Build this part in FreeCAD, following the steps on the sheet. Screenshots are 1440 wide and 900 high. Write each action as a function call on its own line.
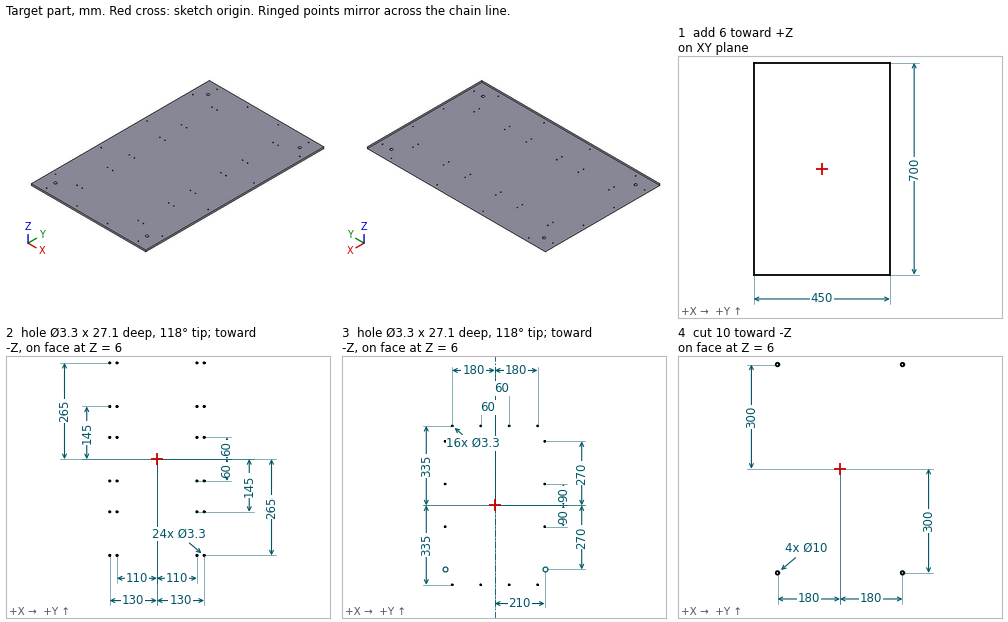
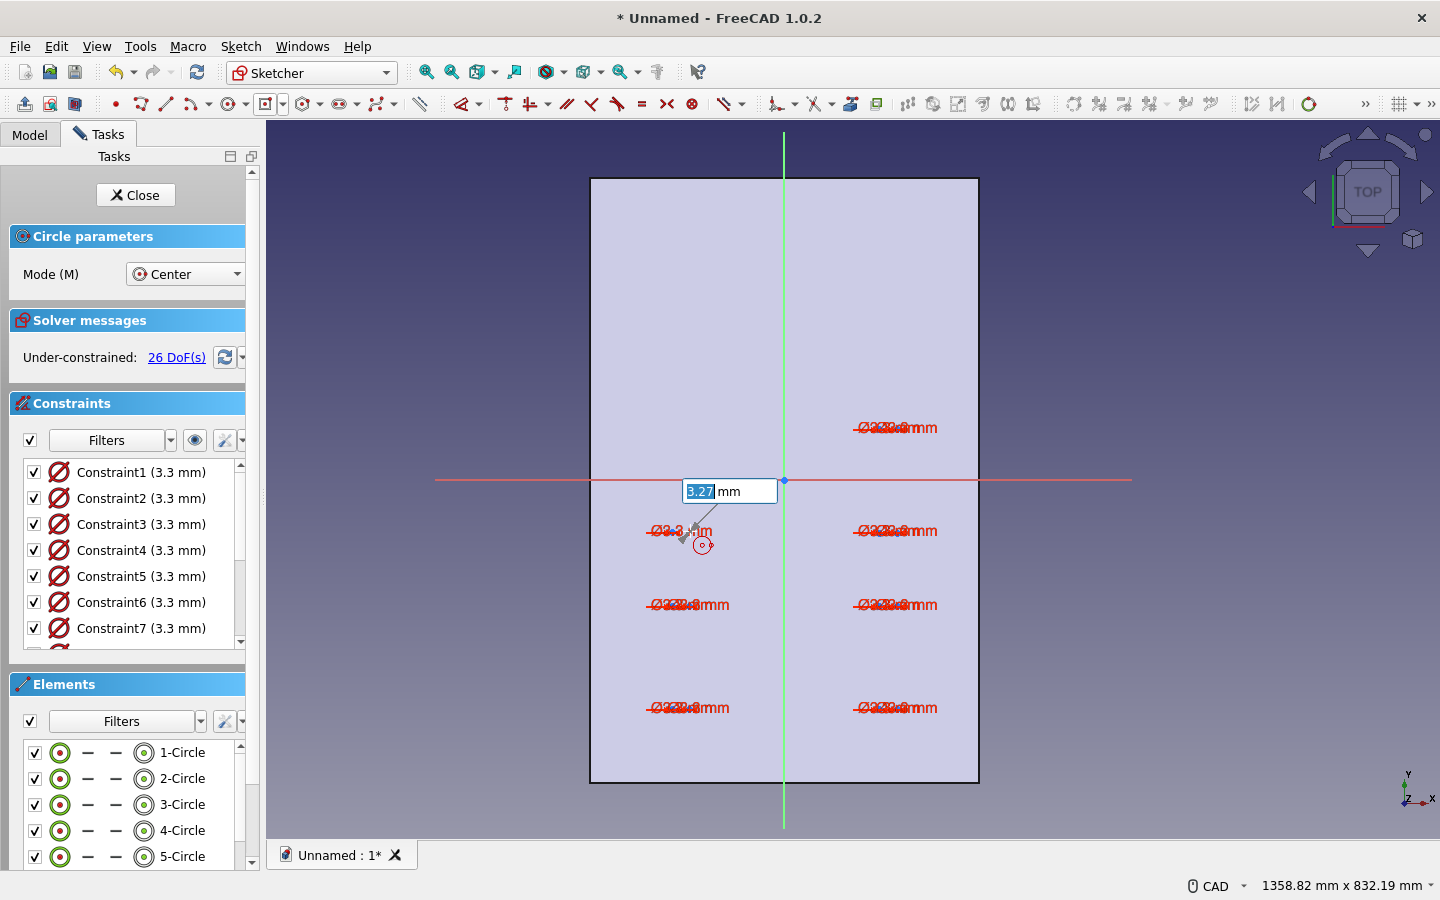
text(3.3)
key(Return)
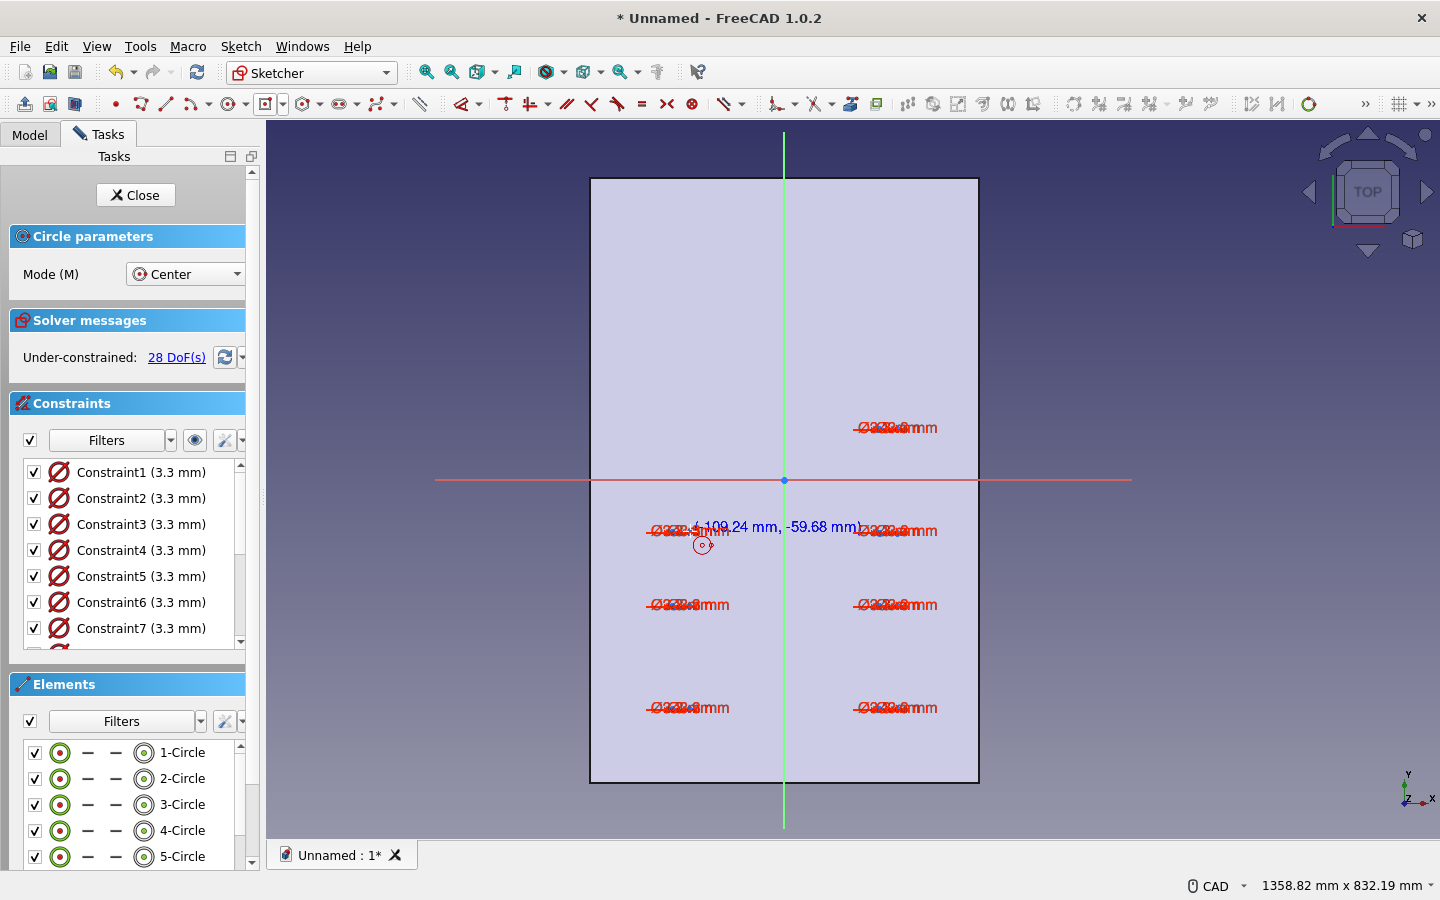
scroll(672, 429, up, 14)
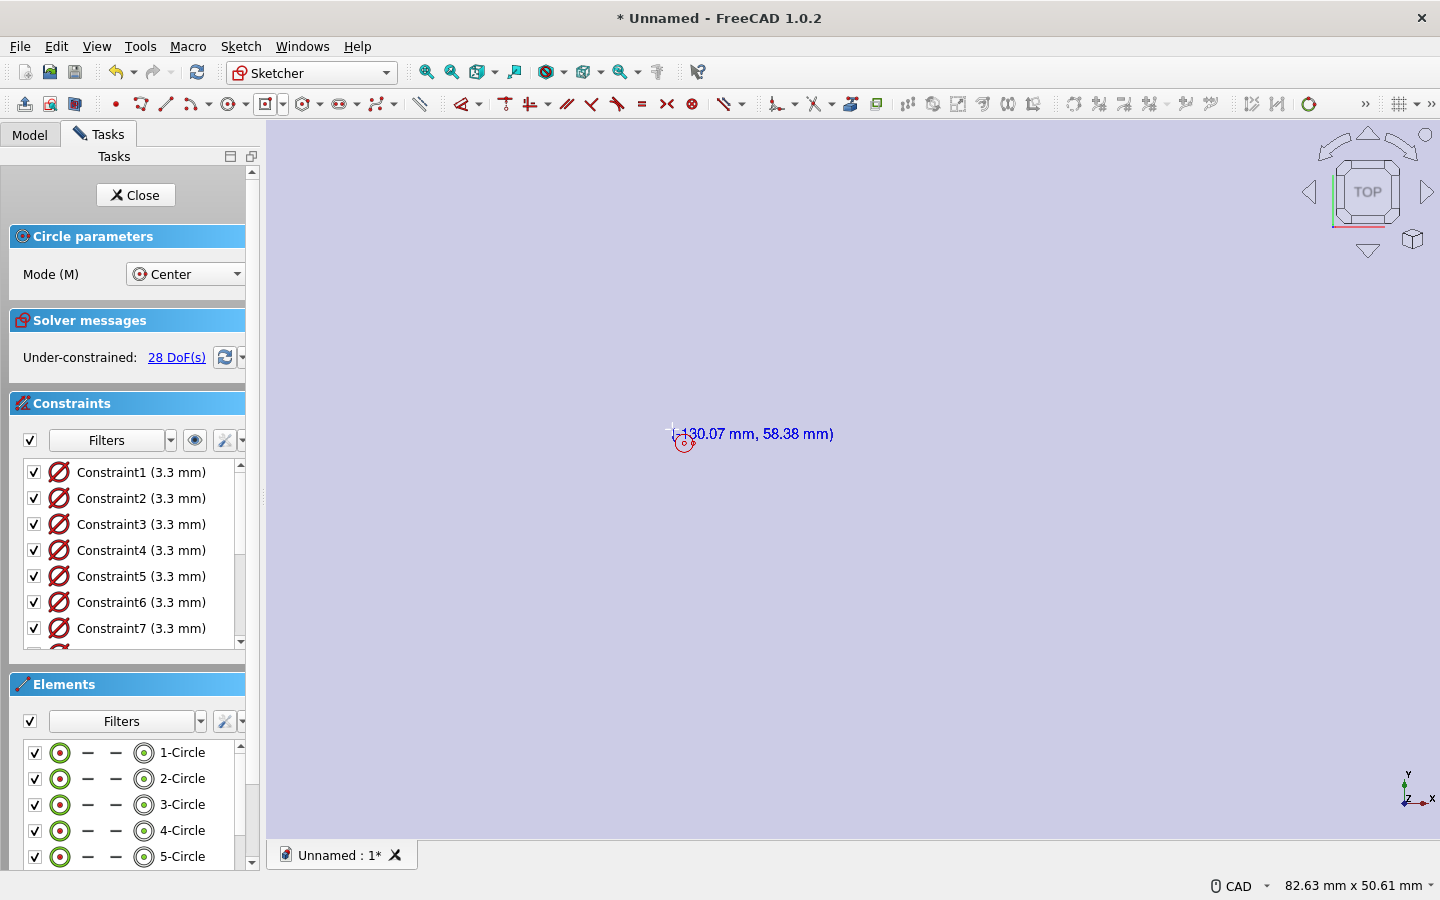
scroll(672, 428, down, 14)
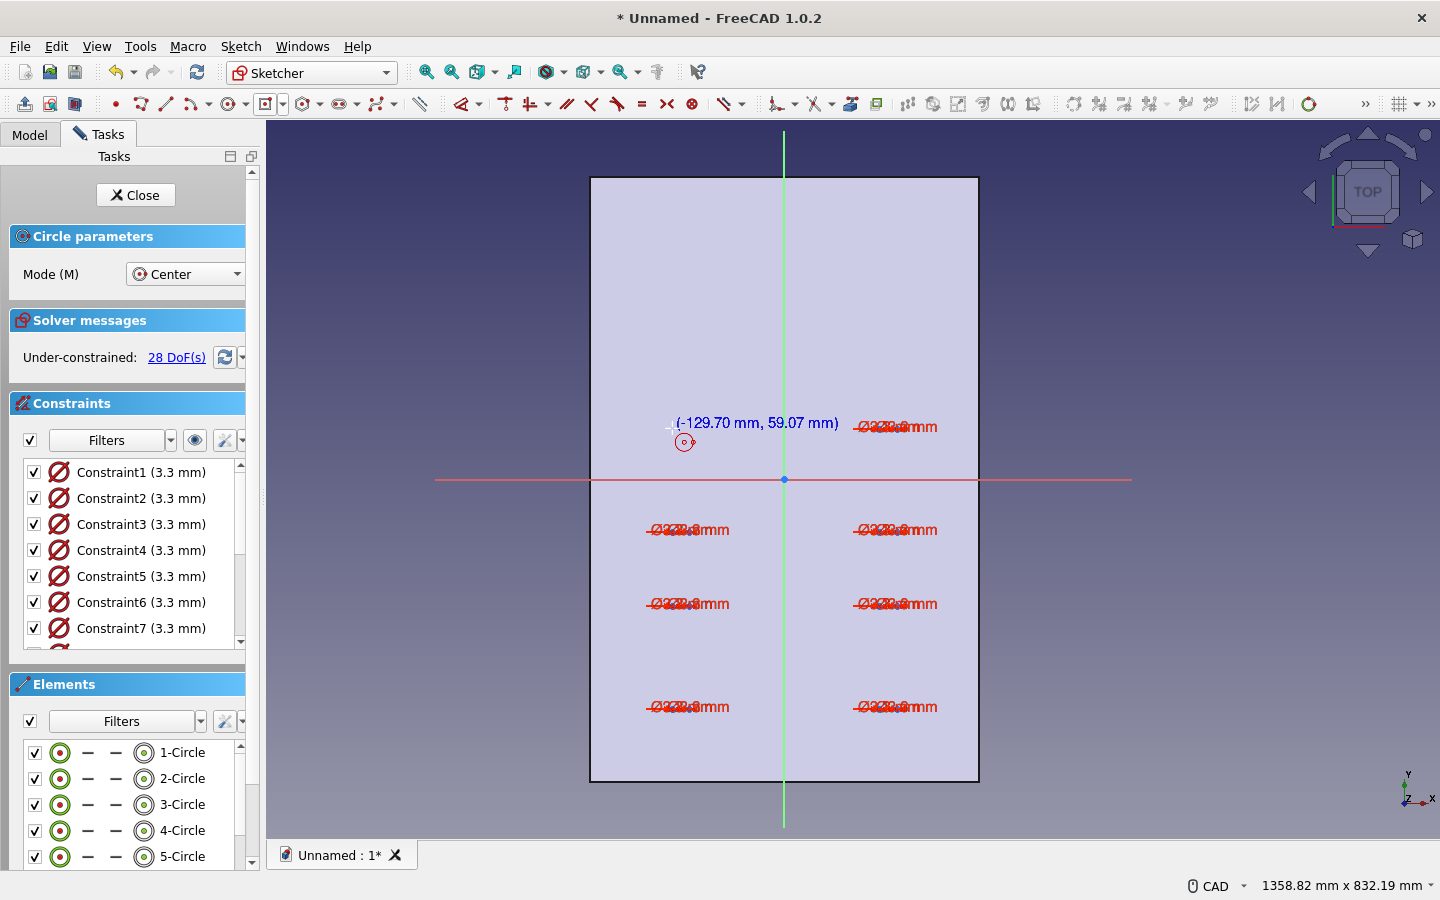
click(672, 428)
move(673, 427)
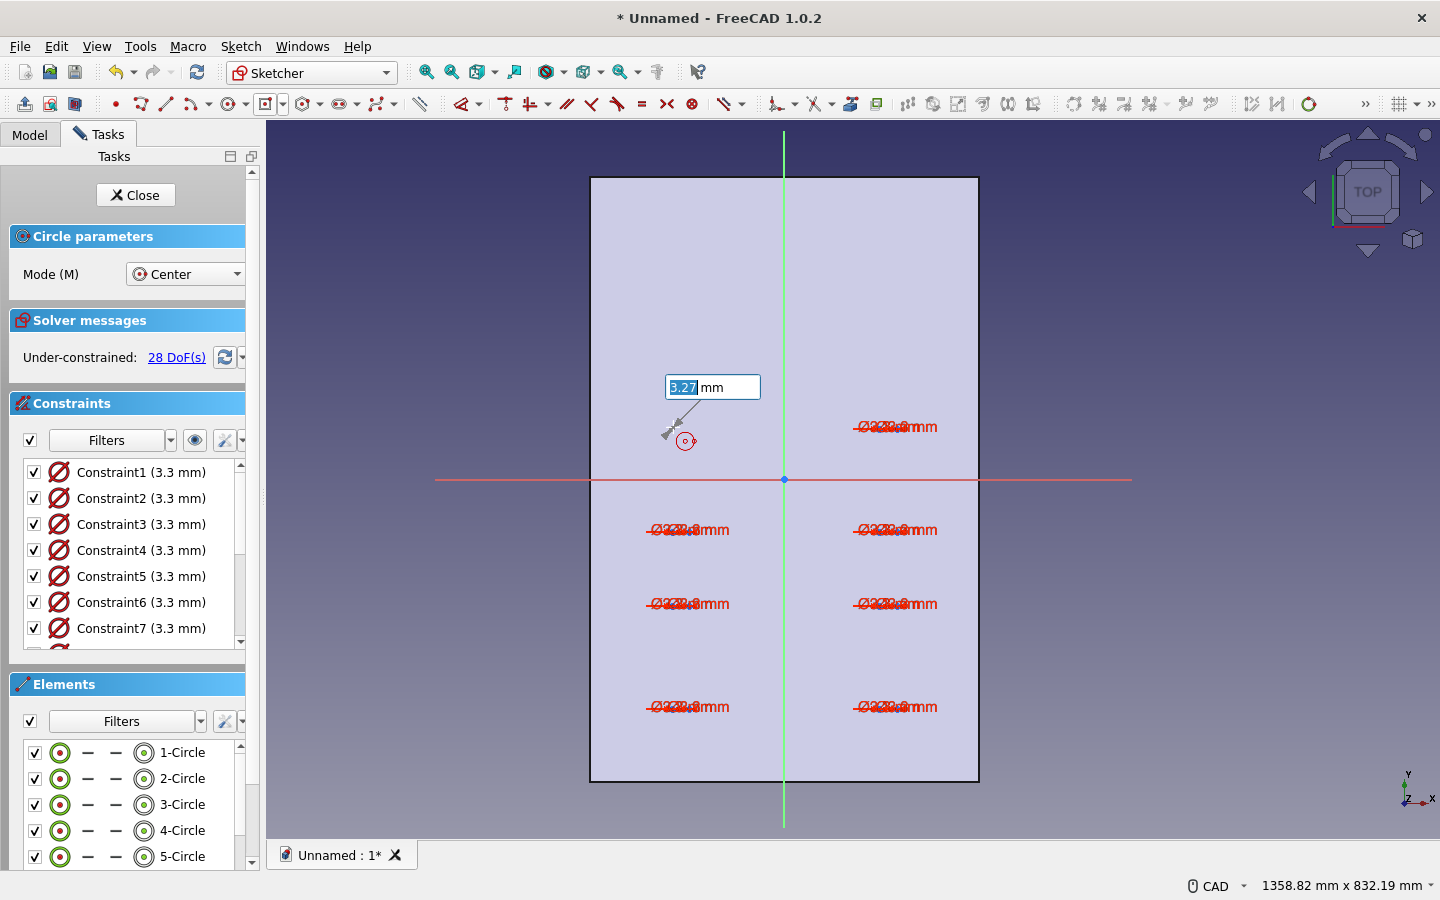
text(3.3)
key(Return)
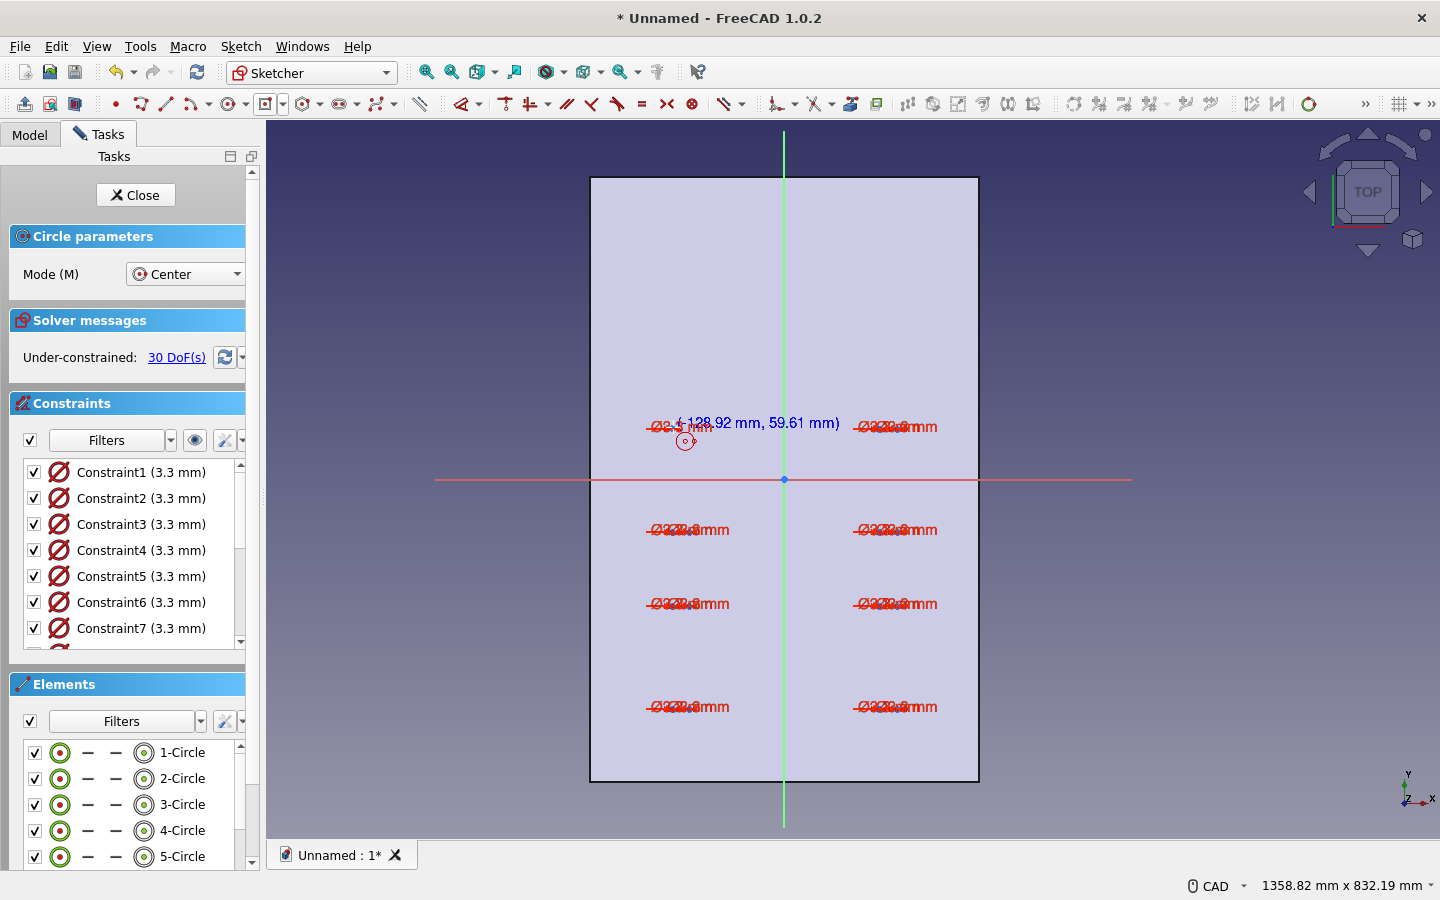
scroll(689, 428, up, 14)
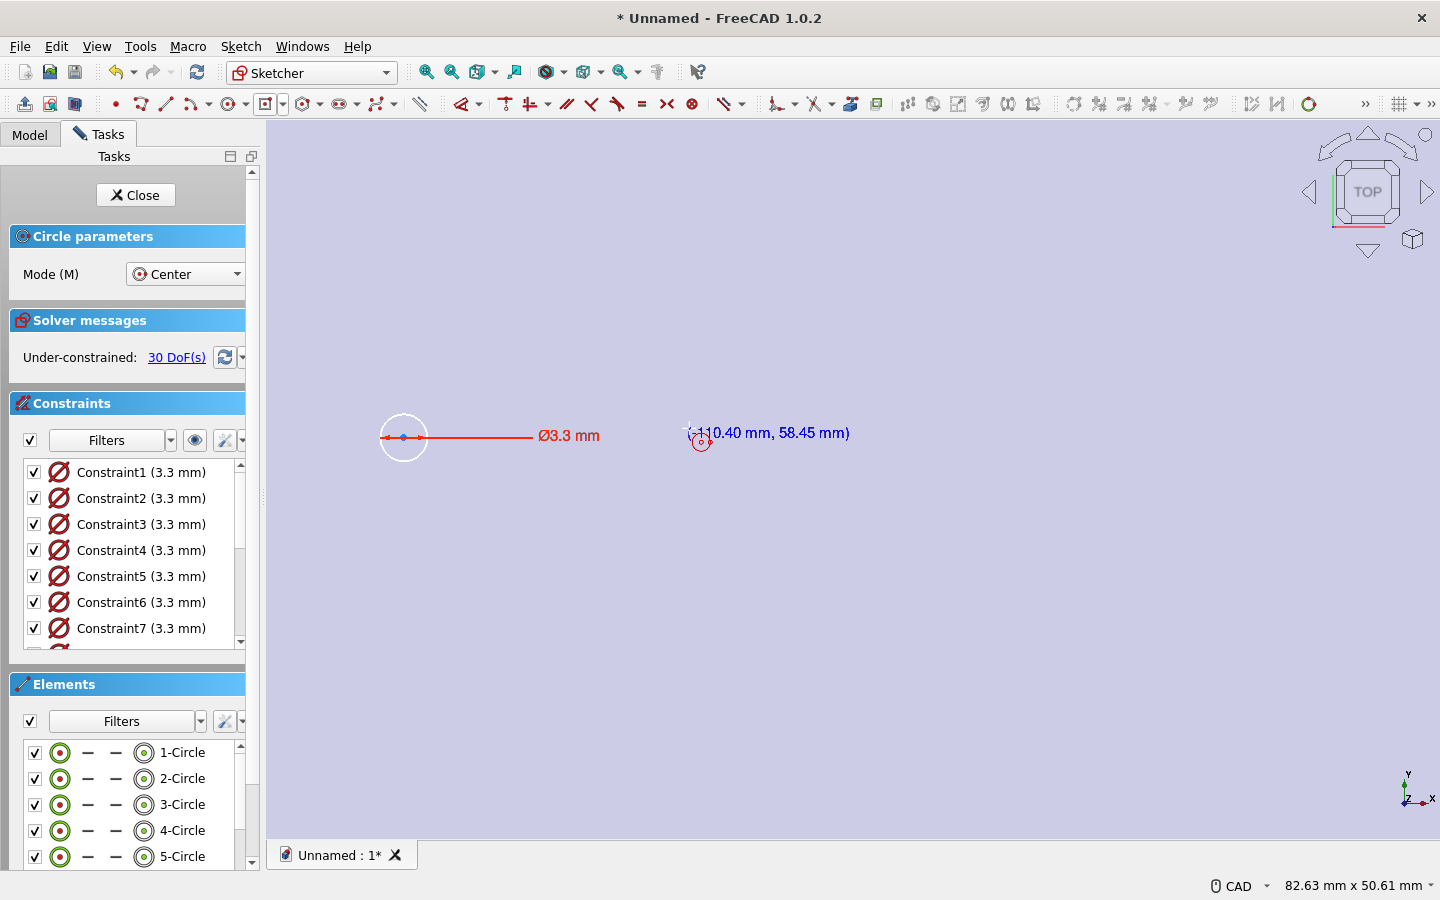
scroll(689, 428, down, 14)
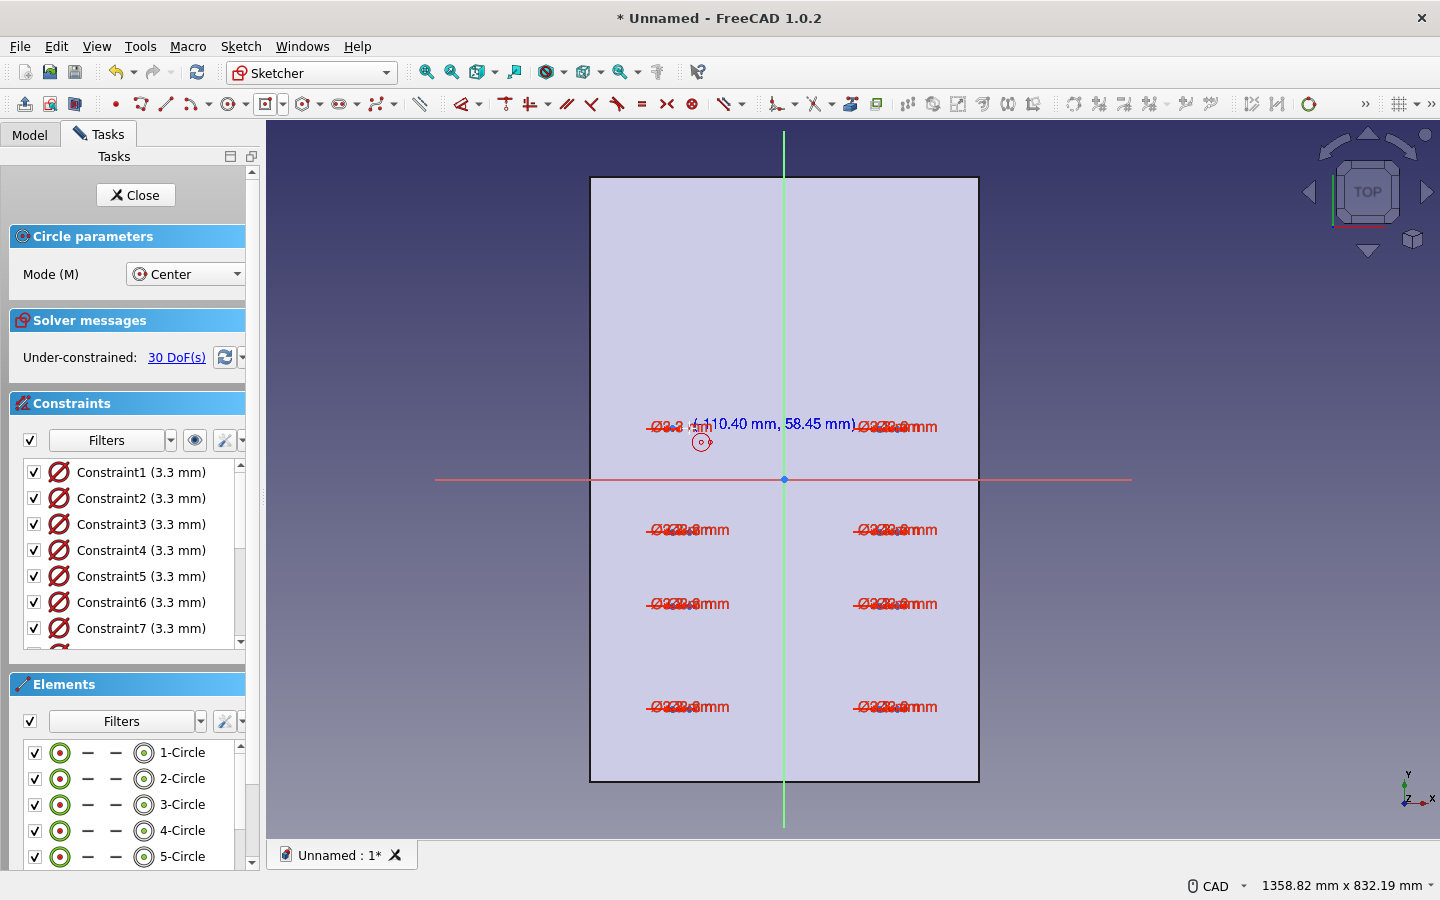
click(689, 428)
move(690, 427)